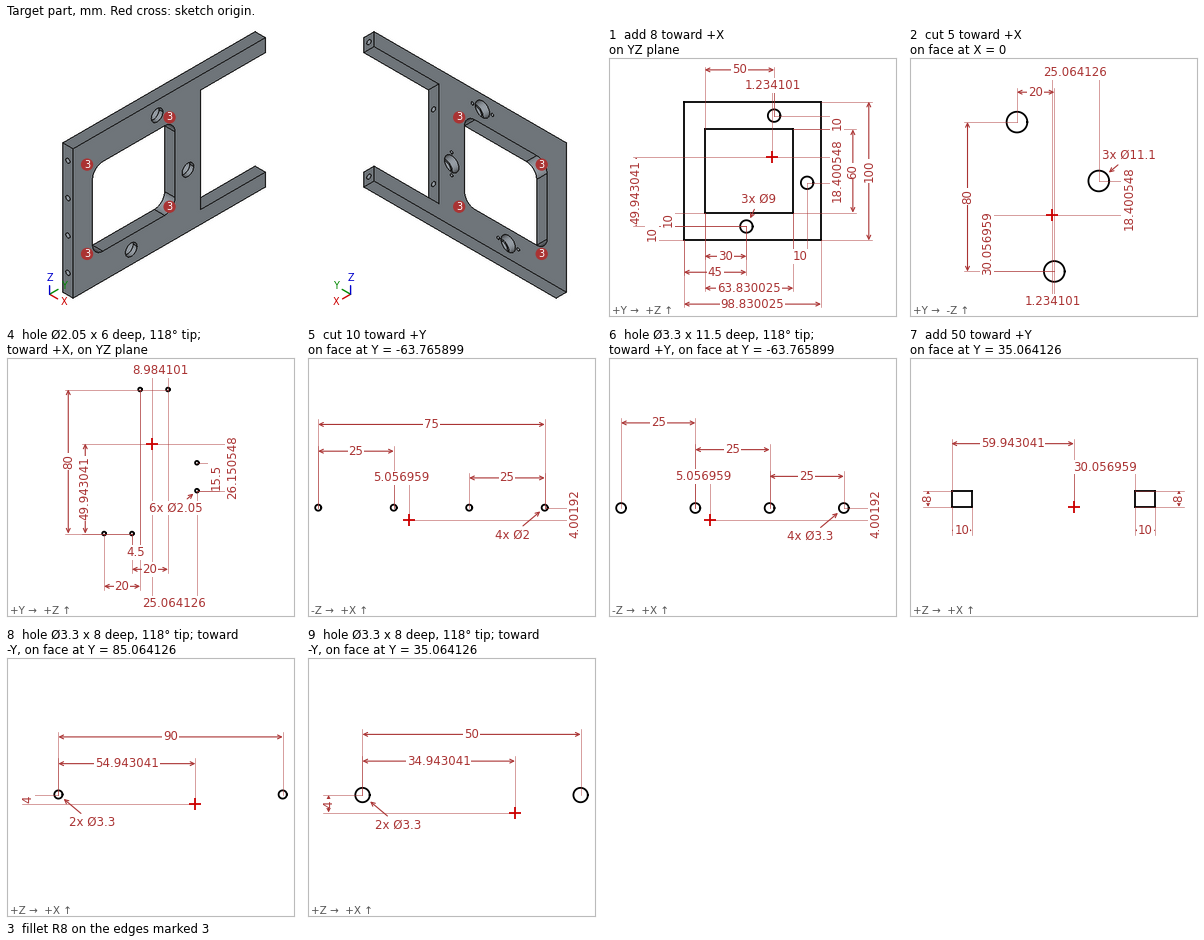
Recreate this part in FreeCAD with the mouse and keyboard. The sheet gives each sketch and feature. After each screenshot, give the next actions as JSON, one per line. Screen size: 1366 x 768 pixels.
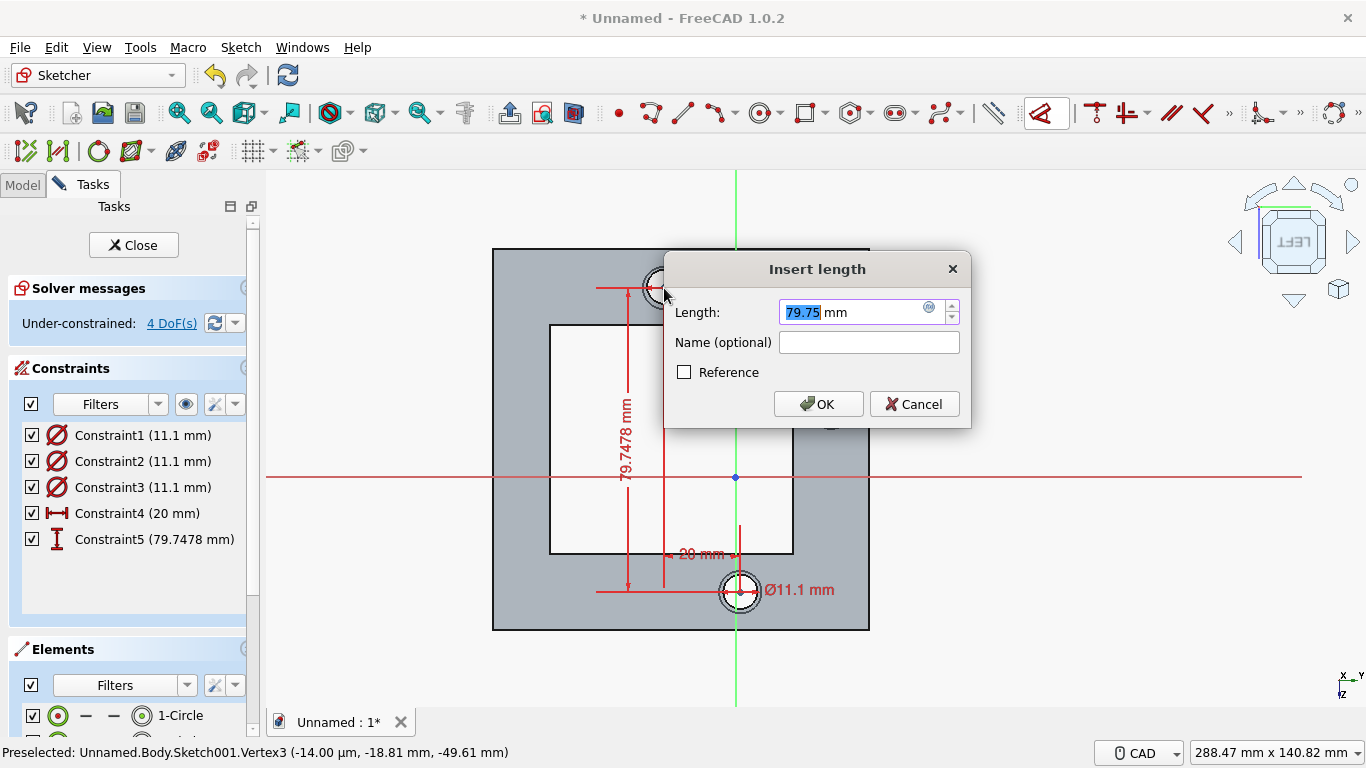
{"action": "type", "text": "80"}
{"action": "key", "text": "Return"}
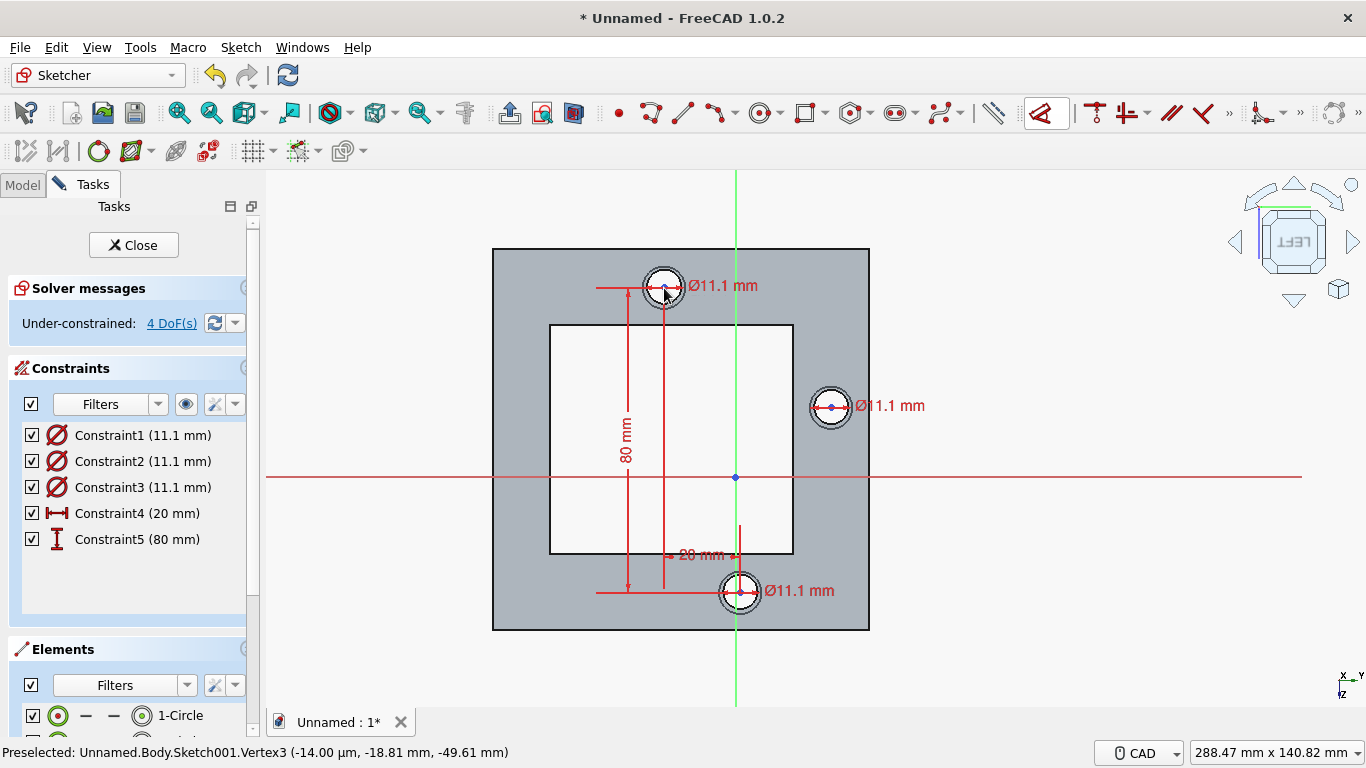
{"action": "scroll", "coordinate": [740, 593], "scroll_direction": "up", "scroll_amount": 11}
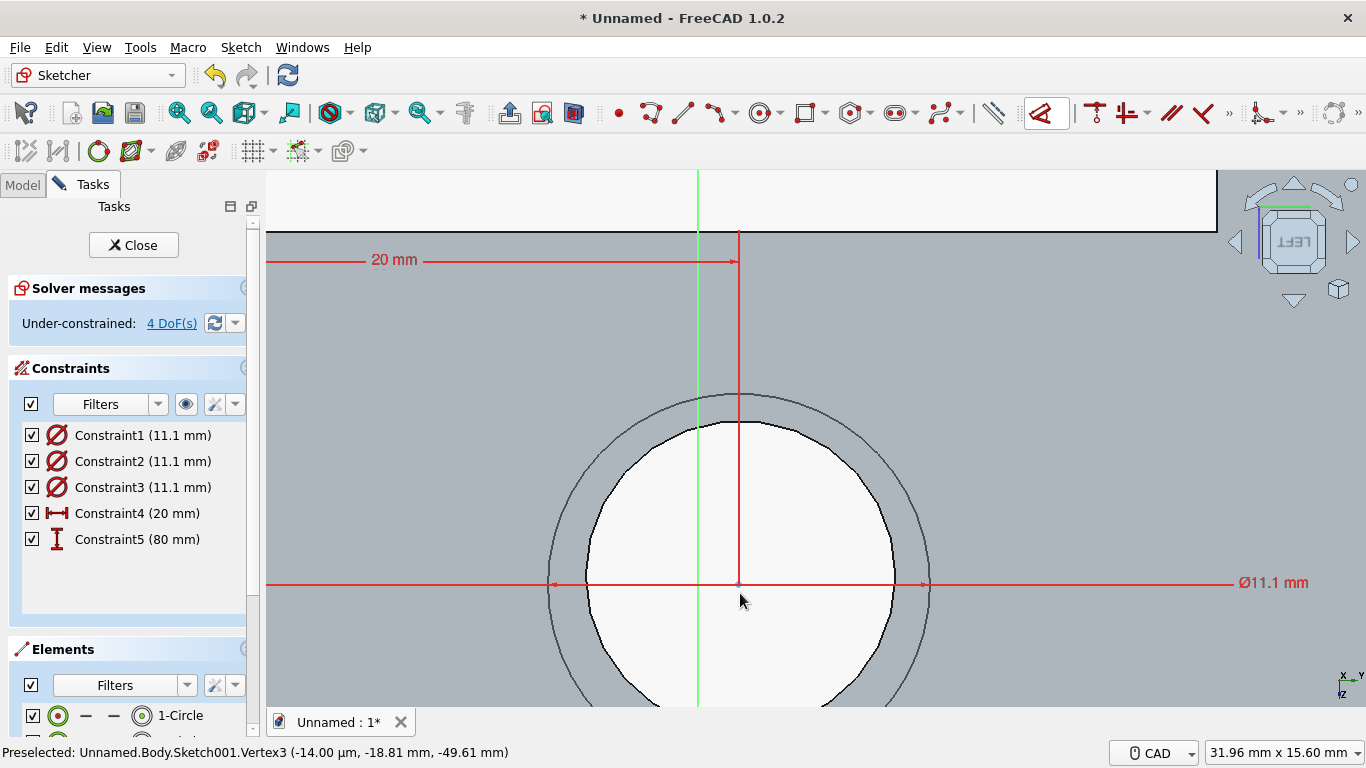
{"action": "left_click", "coordinate": [739, 585]}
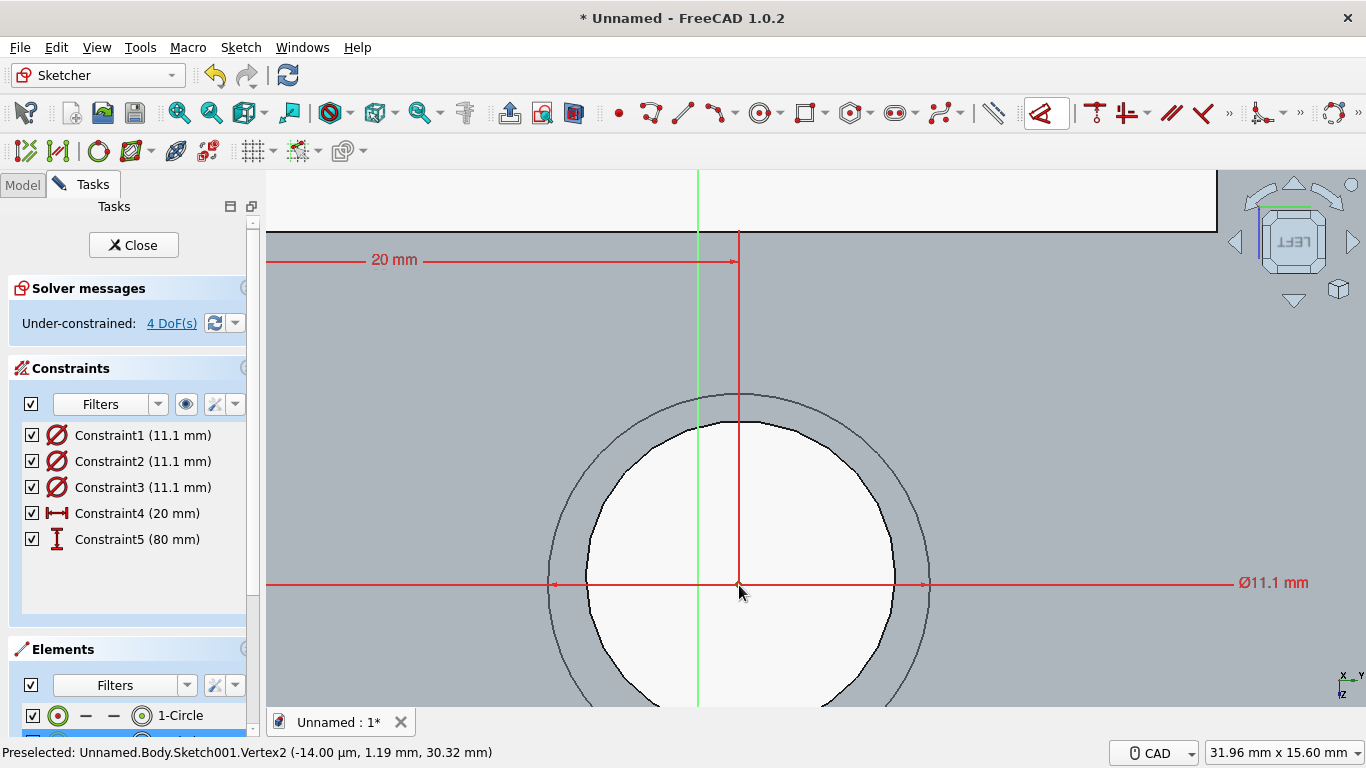
{"action": "left_click", "coordinate": [1064, 114]}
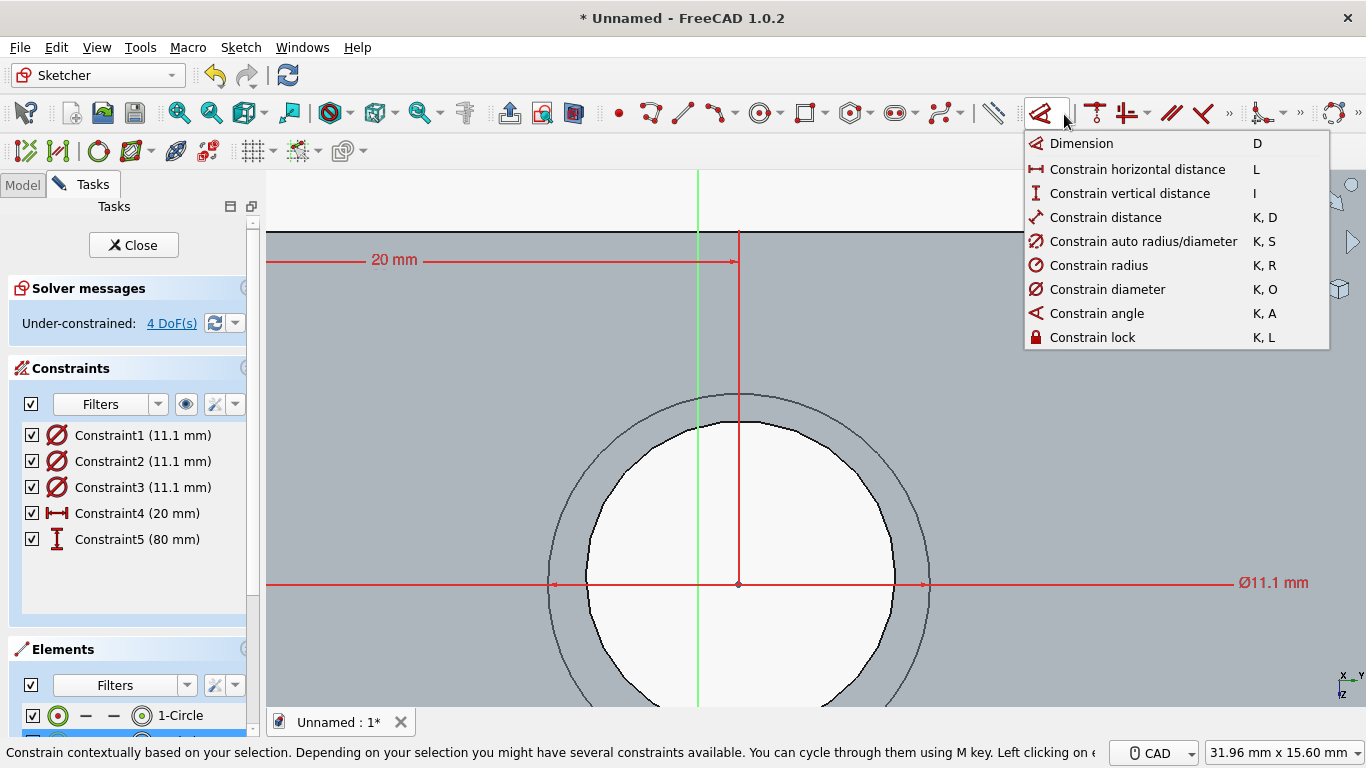
{"action": "left_click", "coordinate": [1177, 169]}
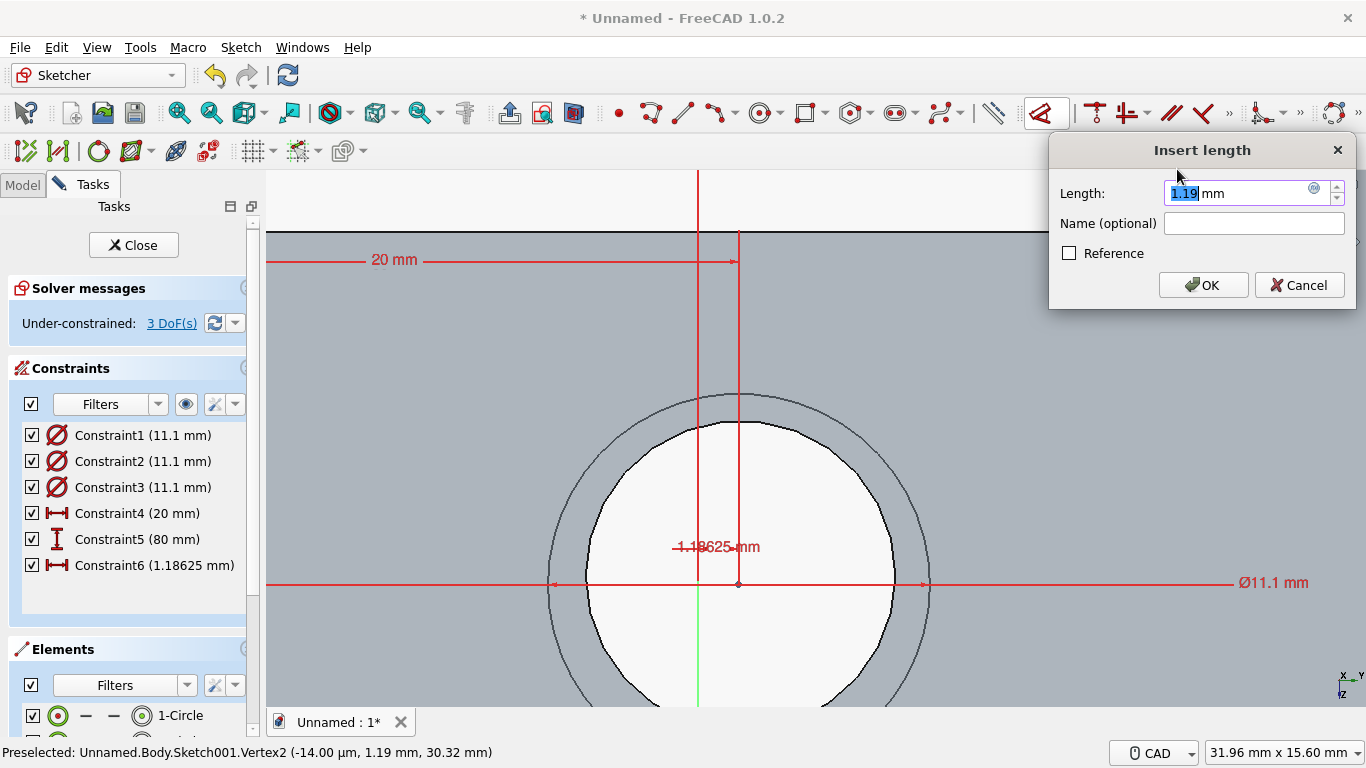
{"action": "type", "text": "1.234101"}
{"action": "key", "text": "Return"}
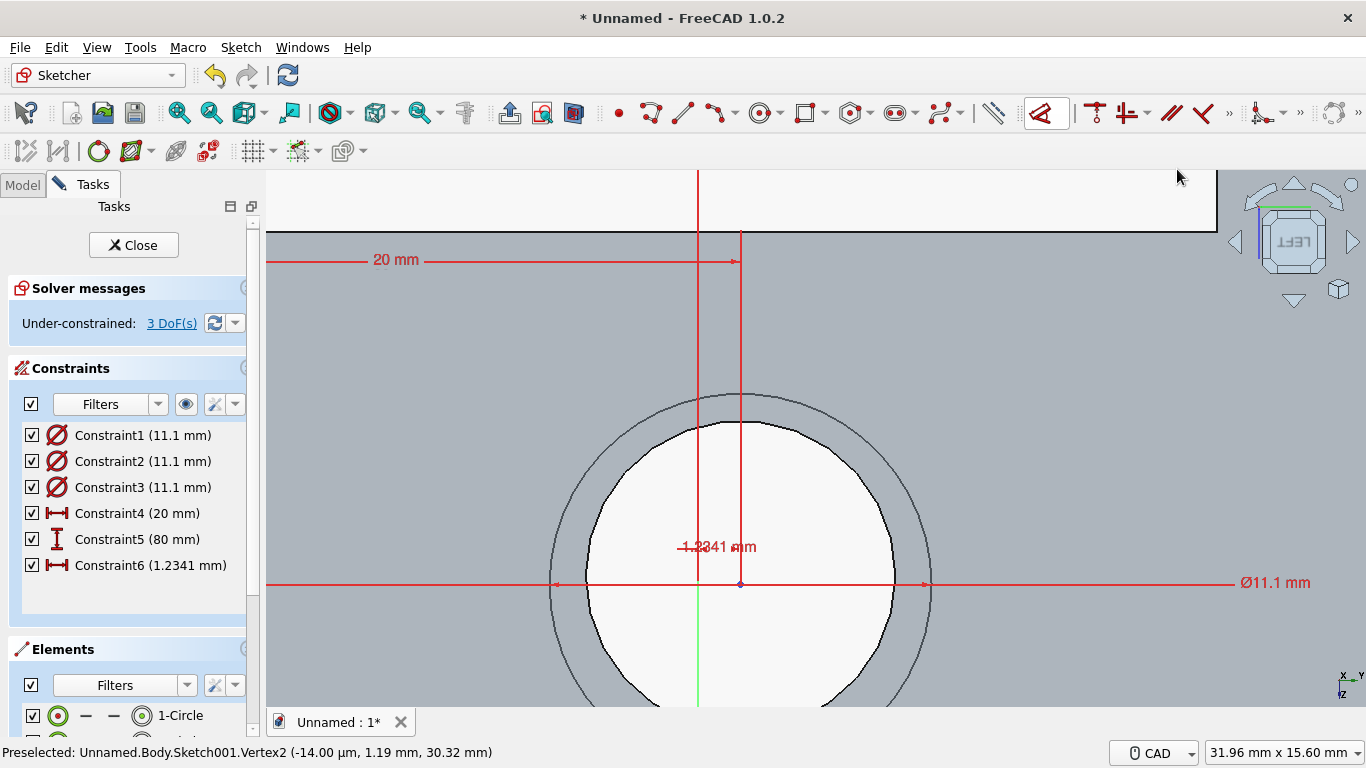
{"action": "scroll", "coordinate": [740, 593], "scroll_direction": "down", "scroll_amount": 11}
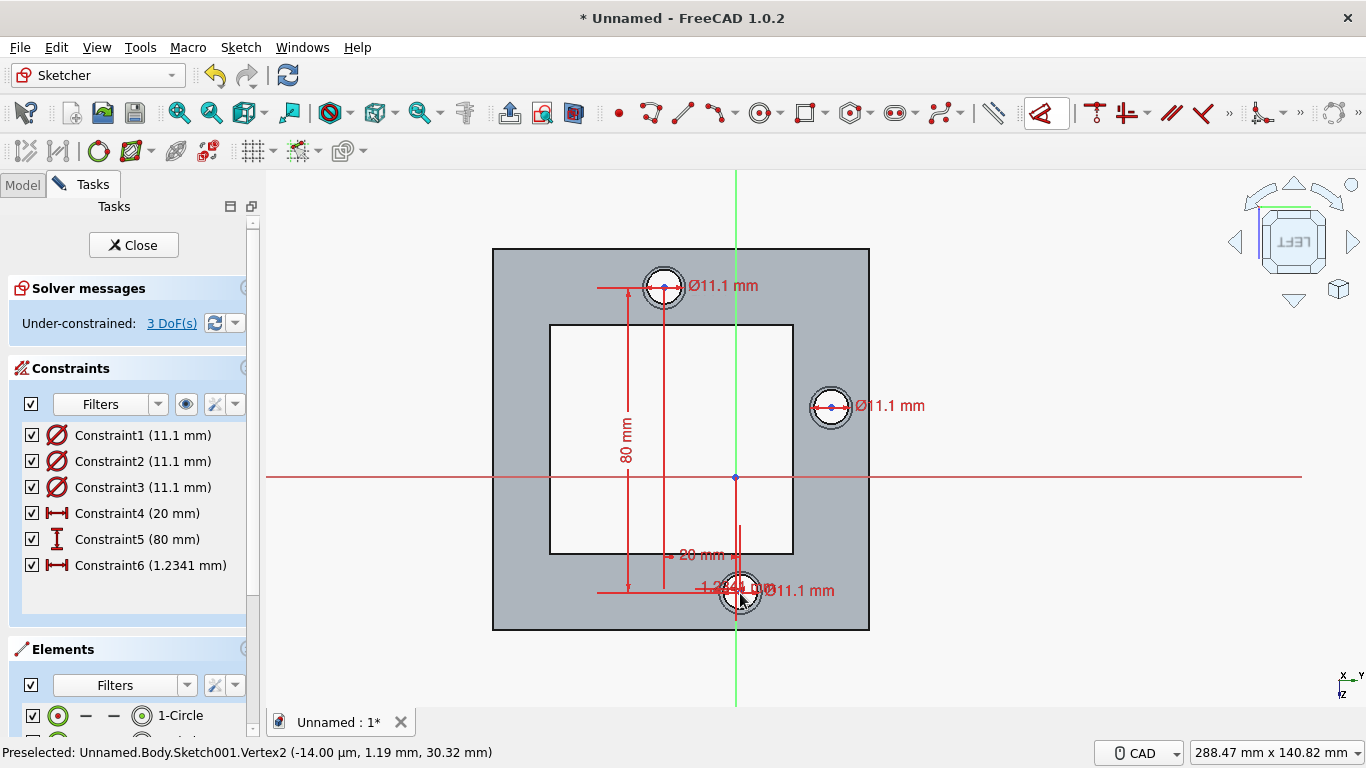
{"action": "left_click", "coordinate": [831, 408]}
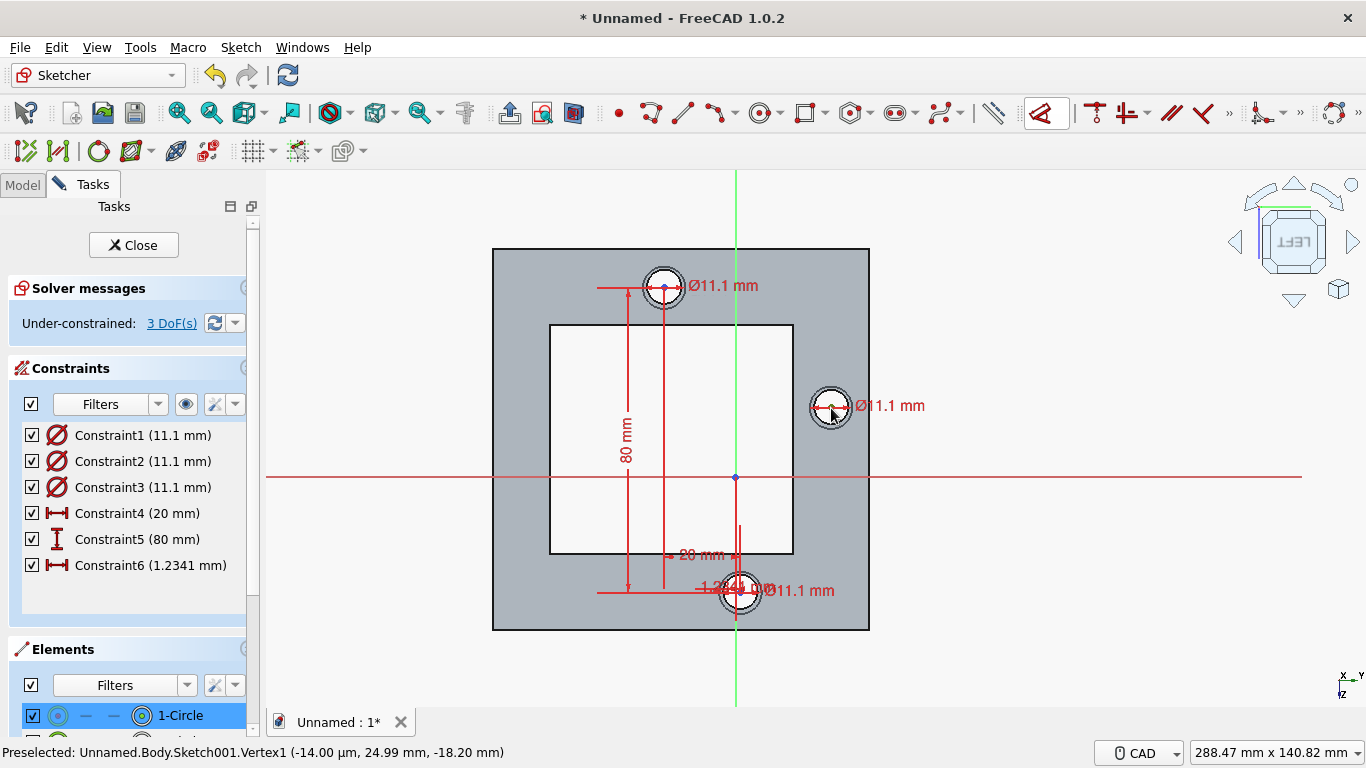
{"action": "left_click", "coordinate": [1064, 114]}